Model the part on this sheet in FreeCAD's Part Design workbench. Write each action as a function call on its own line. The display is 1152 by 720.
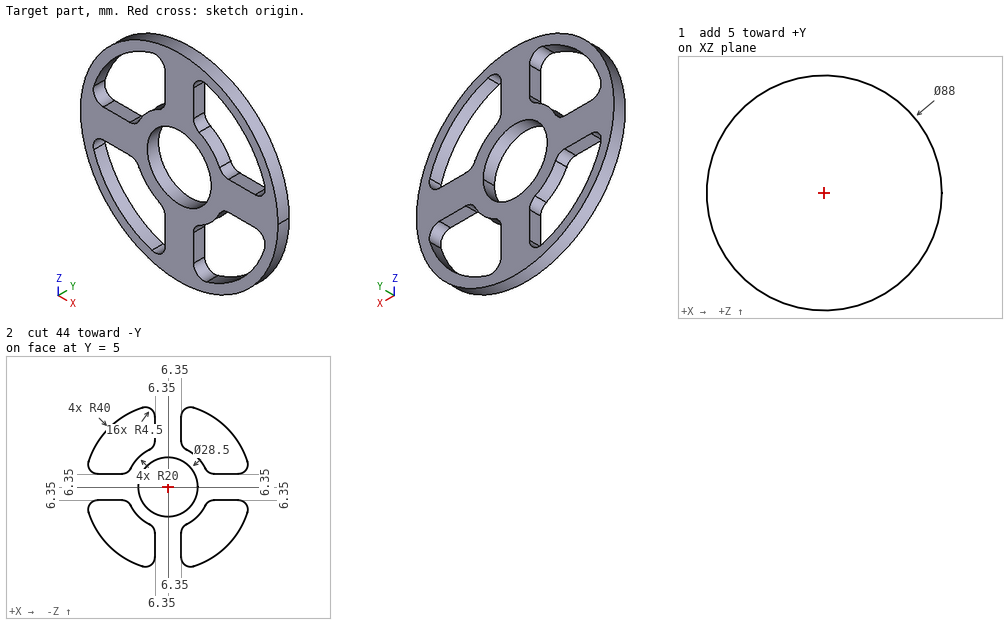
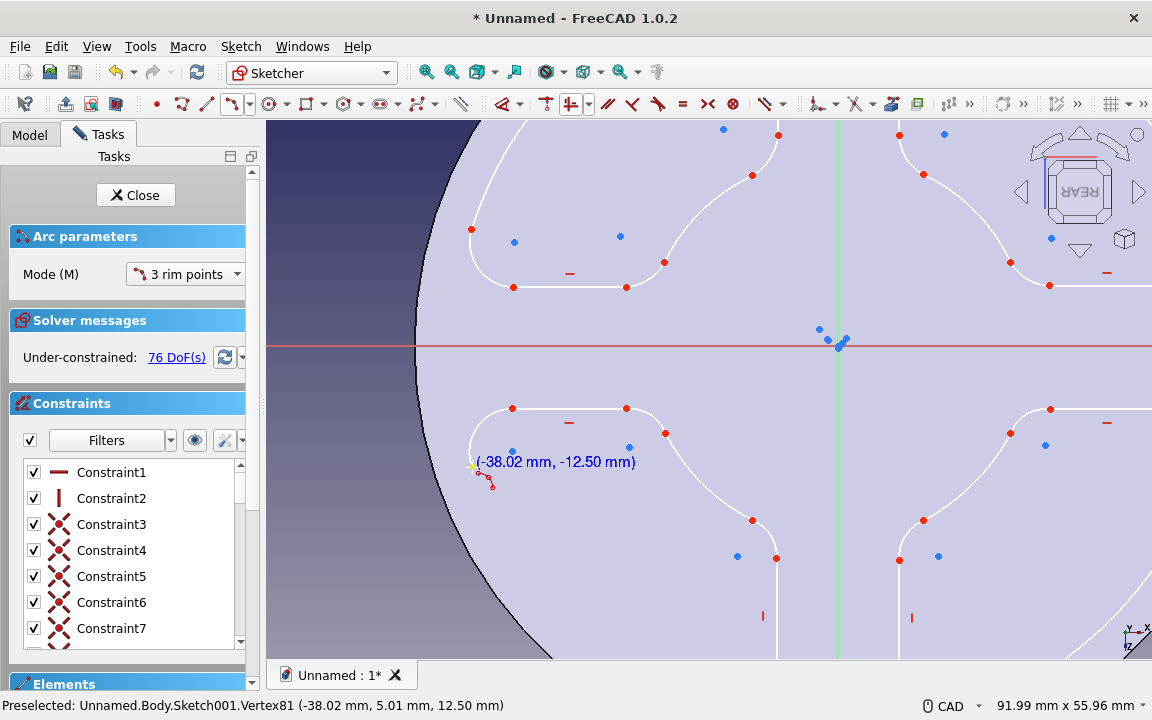
scroll(479, 425, down, 4)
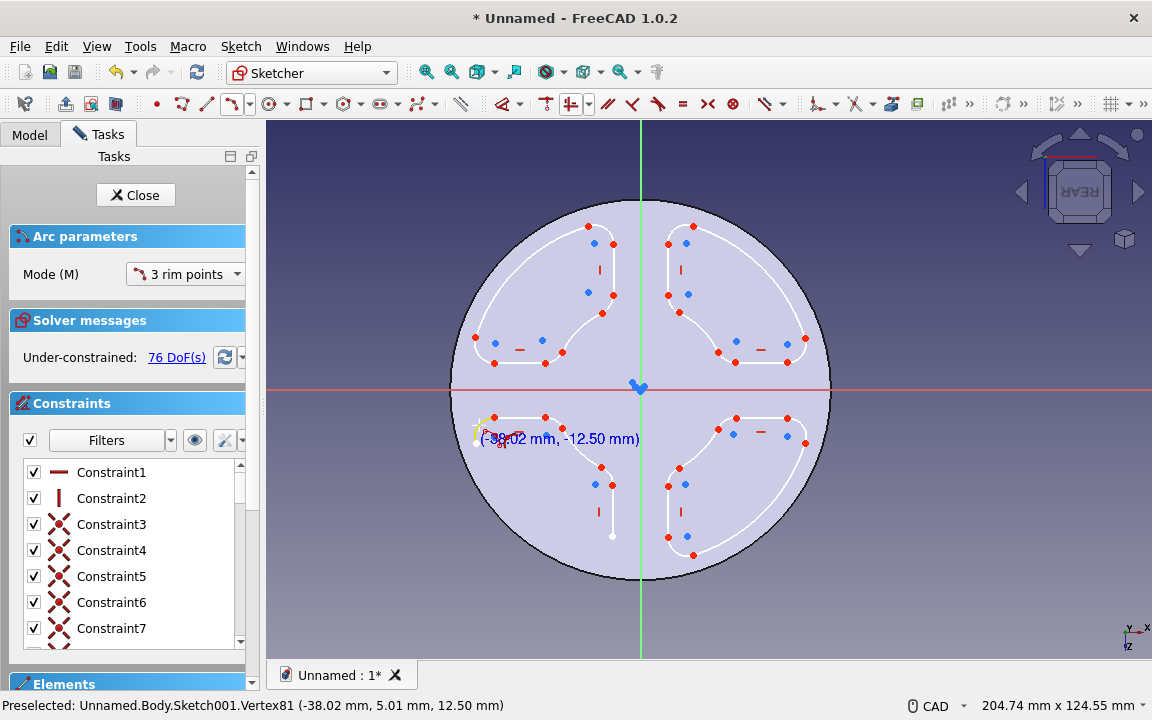
click(588, 555)
click(518, 512)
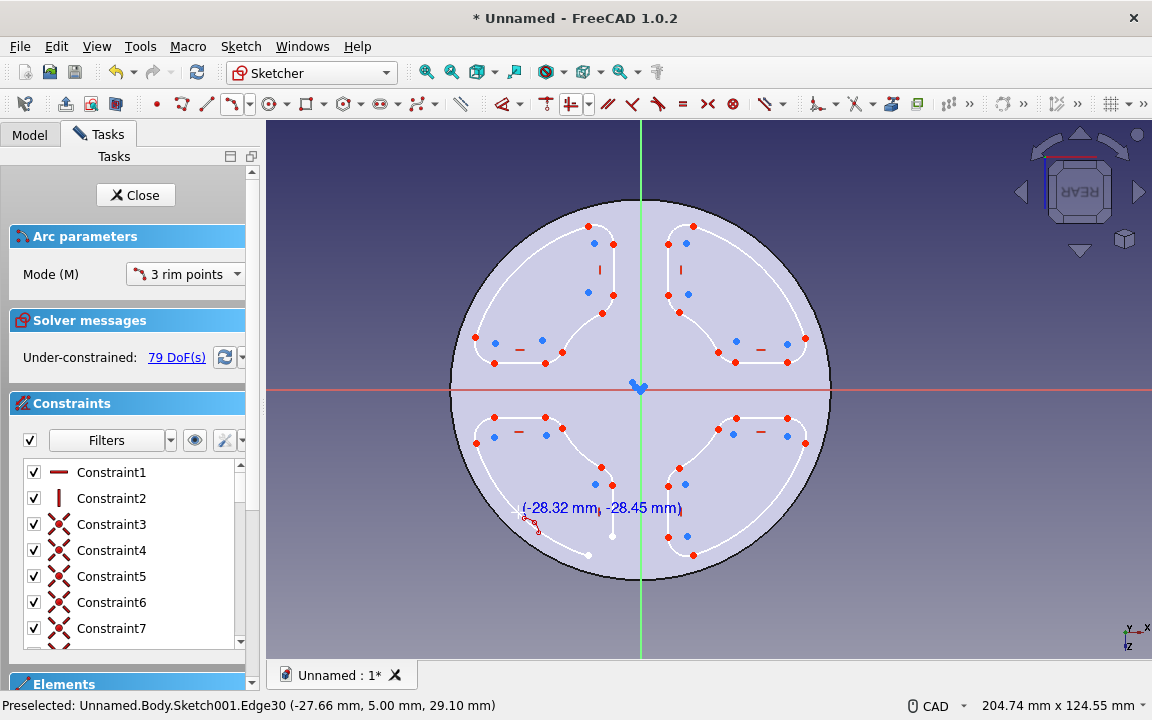
click(588, 556)
click(613, 537)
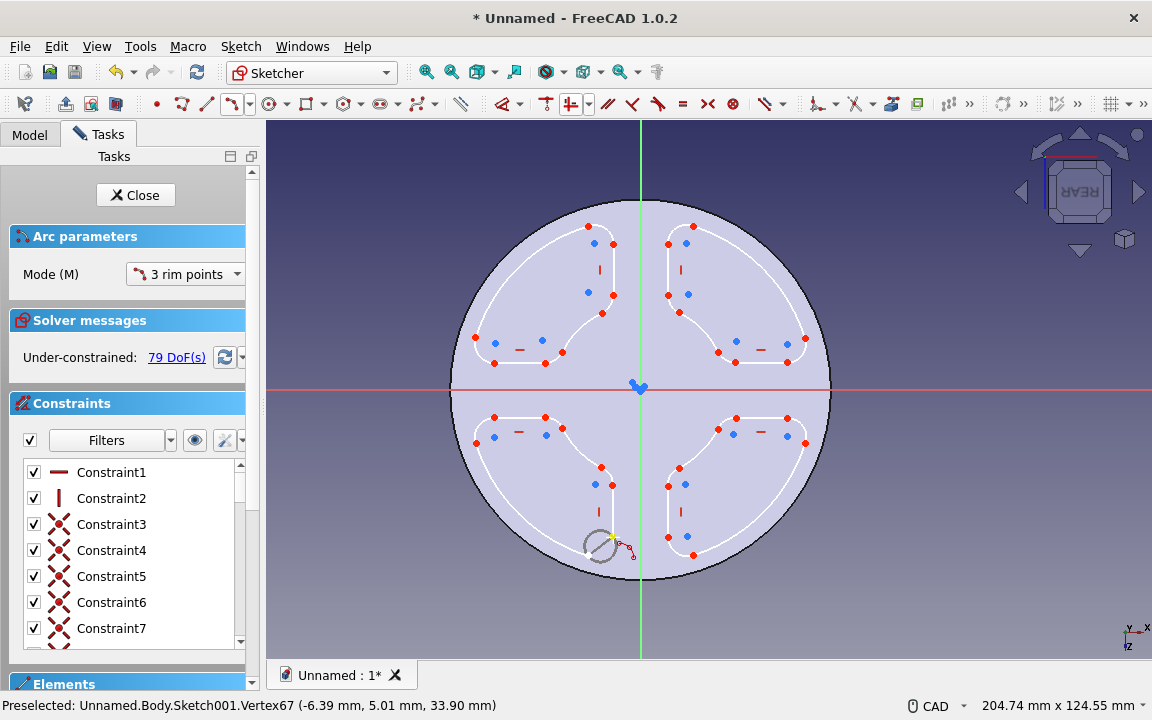
scroll(605, 552, up, 4)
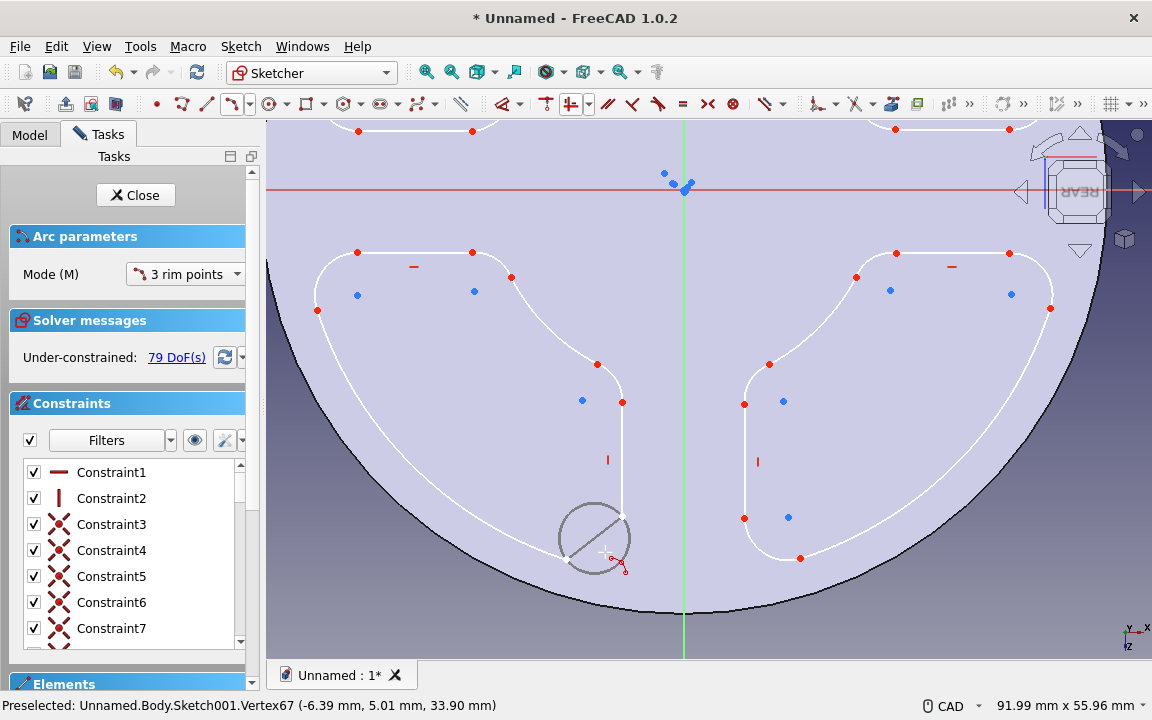
click(605, 551)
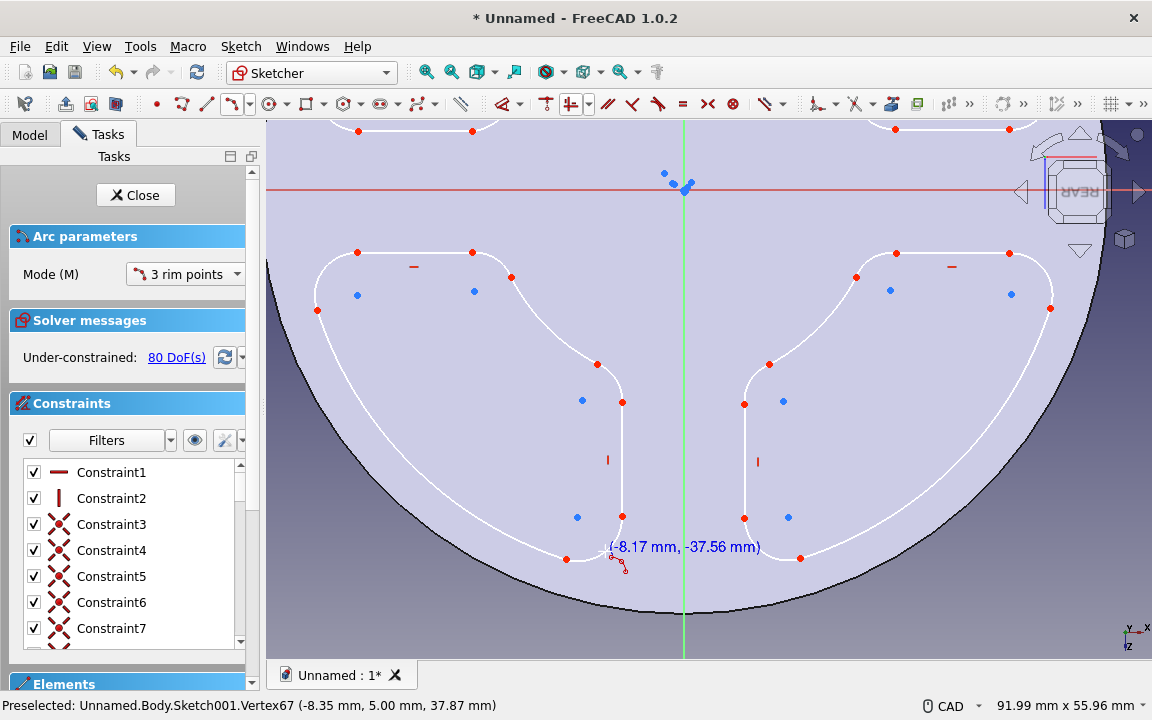
key(g)
key(c)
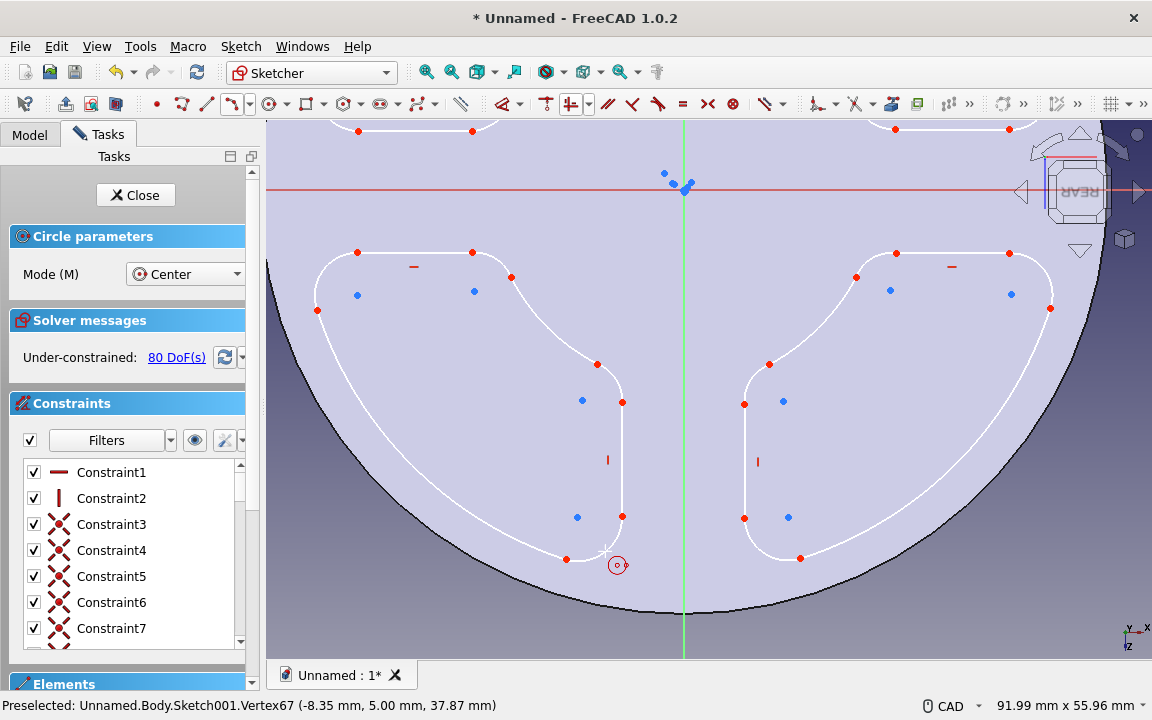
click(684, 190)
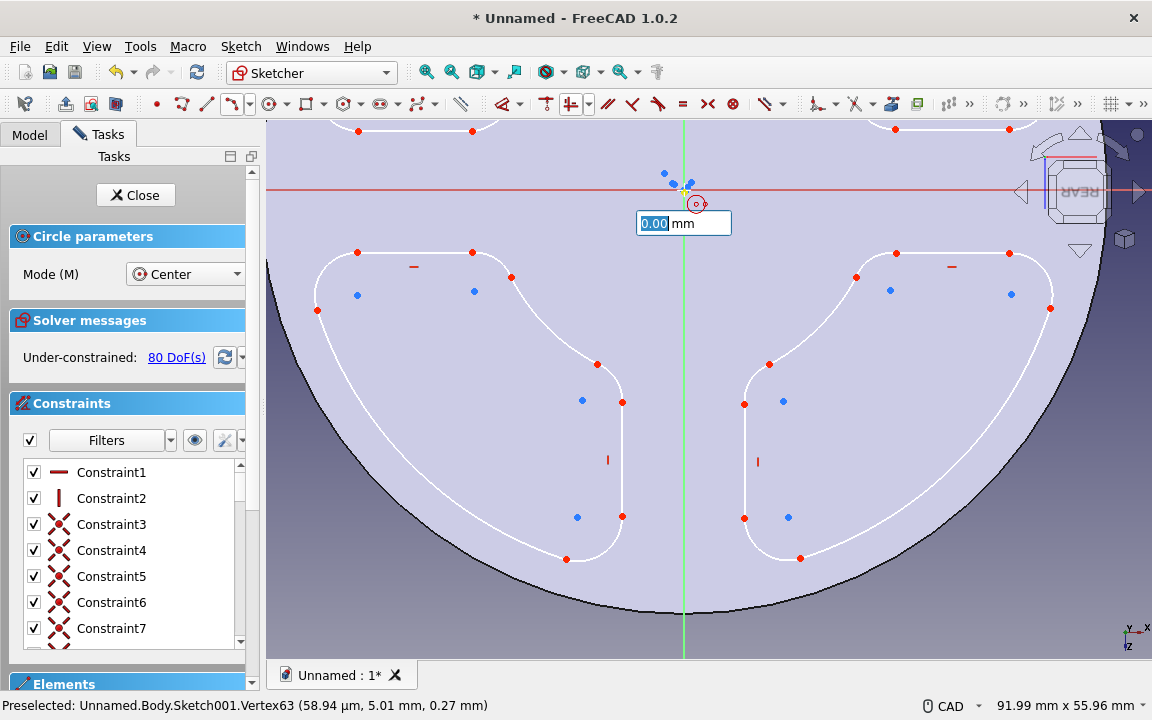
scroll(605, 552, down, 4)
move(684, 346)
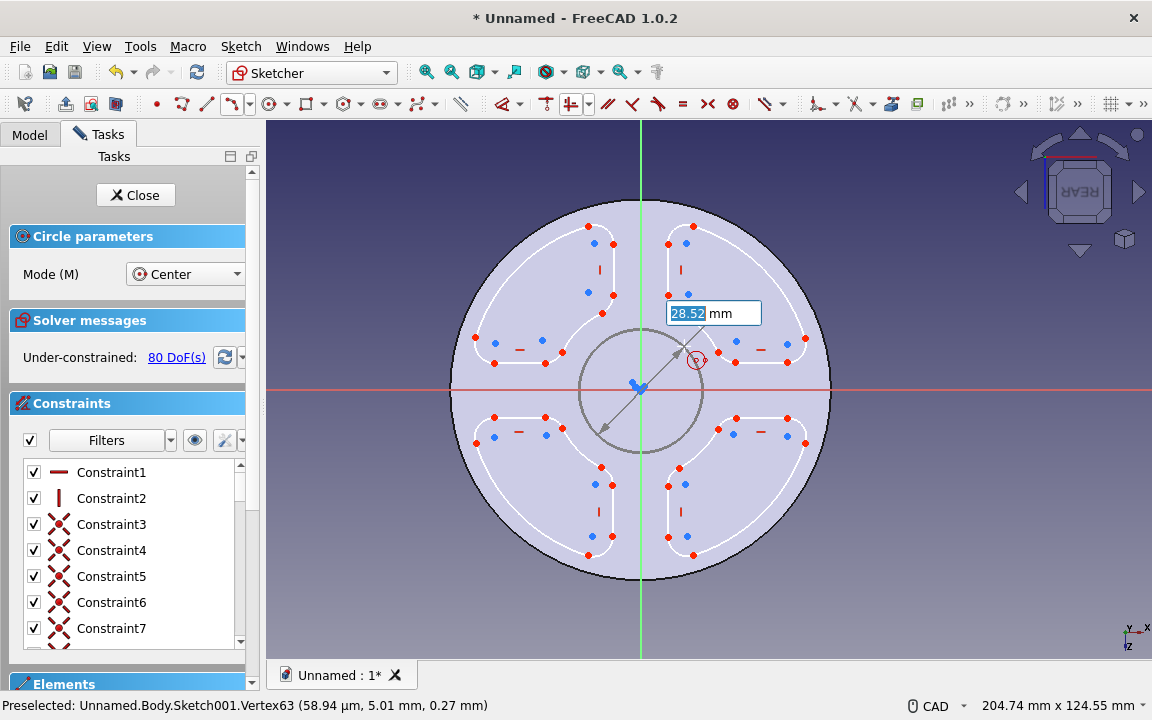
text(28.5)
key(Return)
key(Escape)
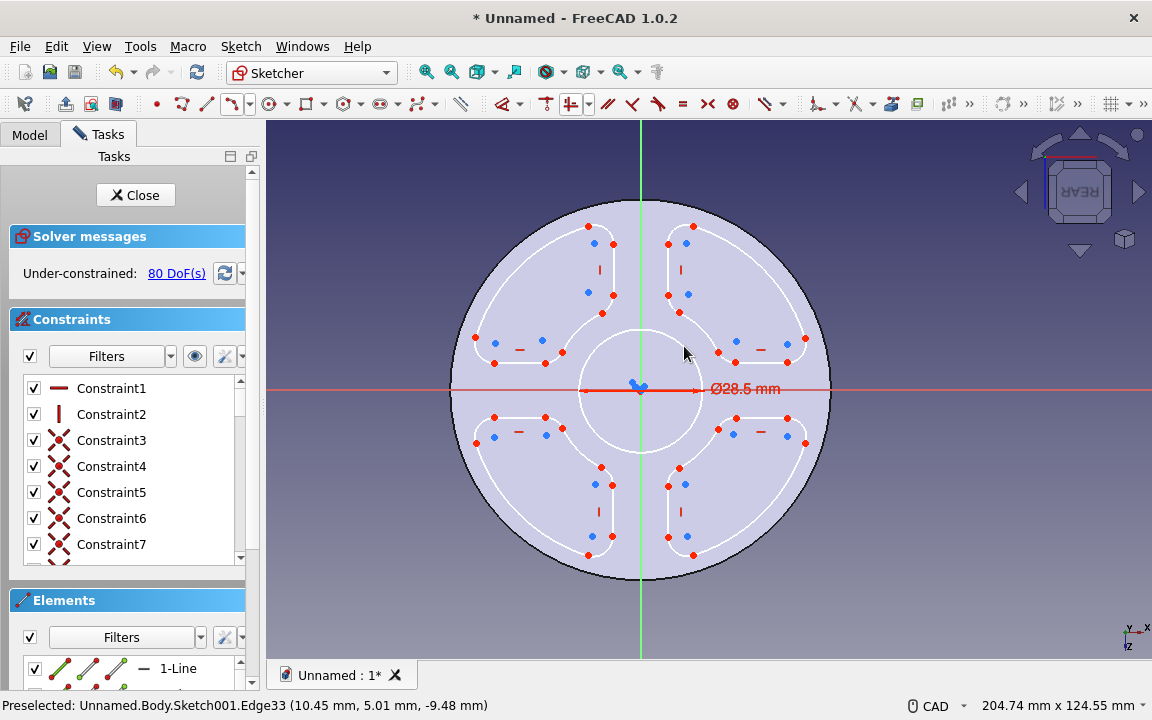
click(510, 363)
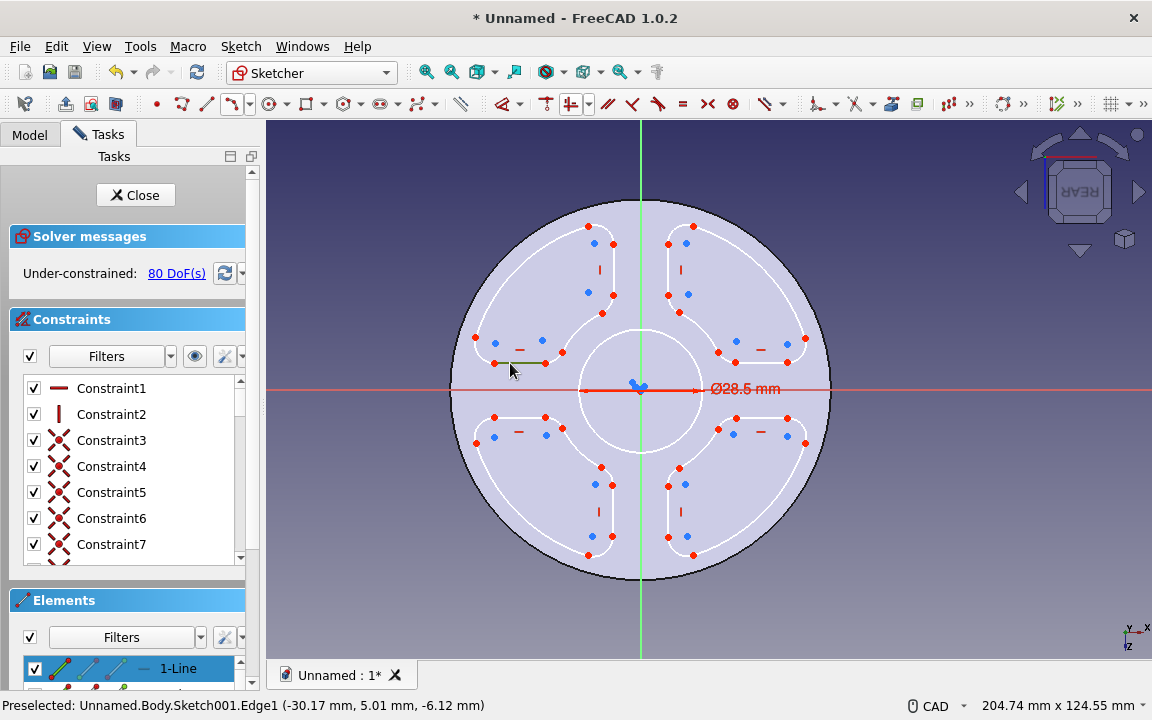
scroll(555, 360, up, 2)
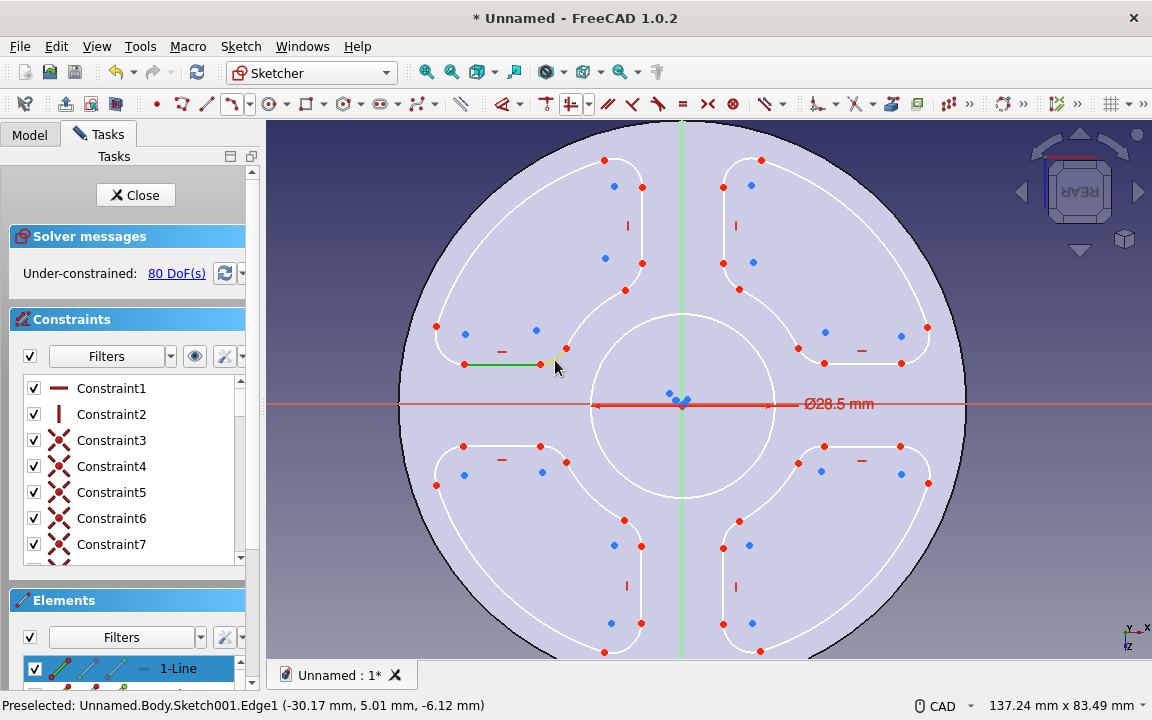
click(555, 360)